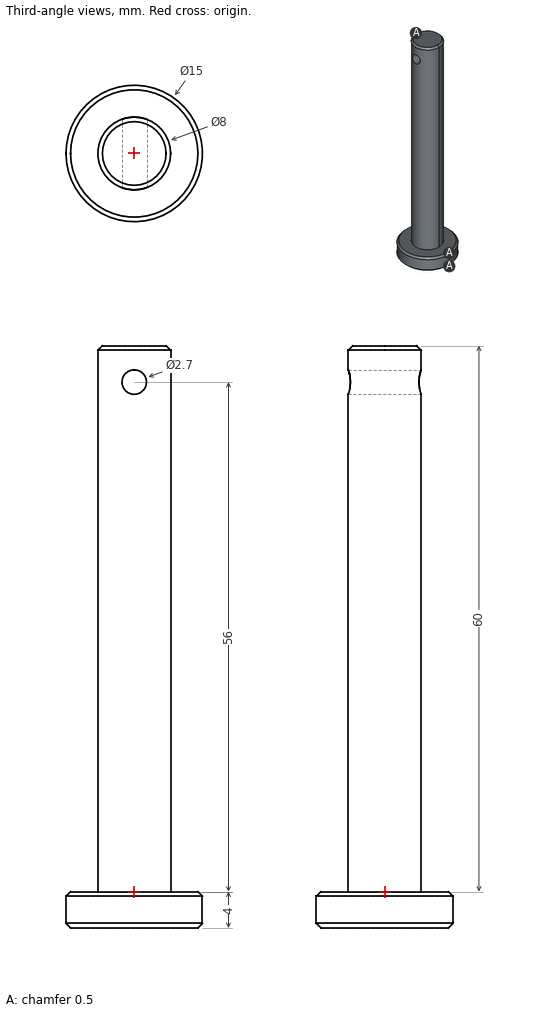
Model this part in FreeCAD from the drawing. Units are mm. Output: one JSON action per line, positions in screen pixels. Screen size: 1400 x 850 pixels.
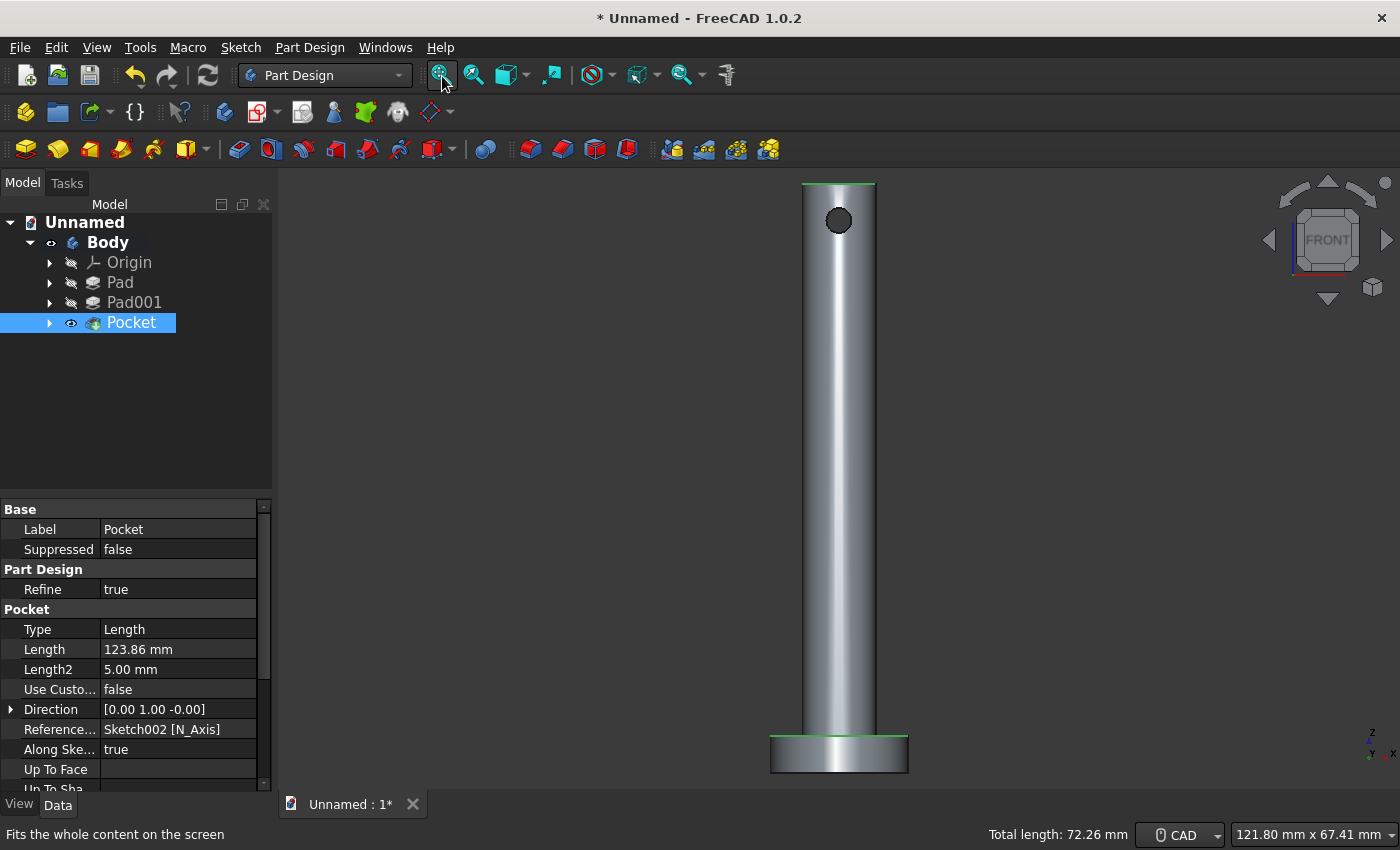
{"action": "key", "text": "3"}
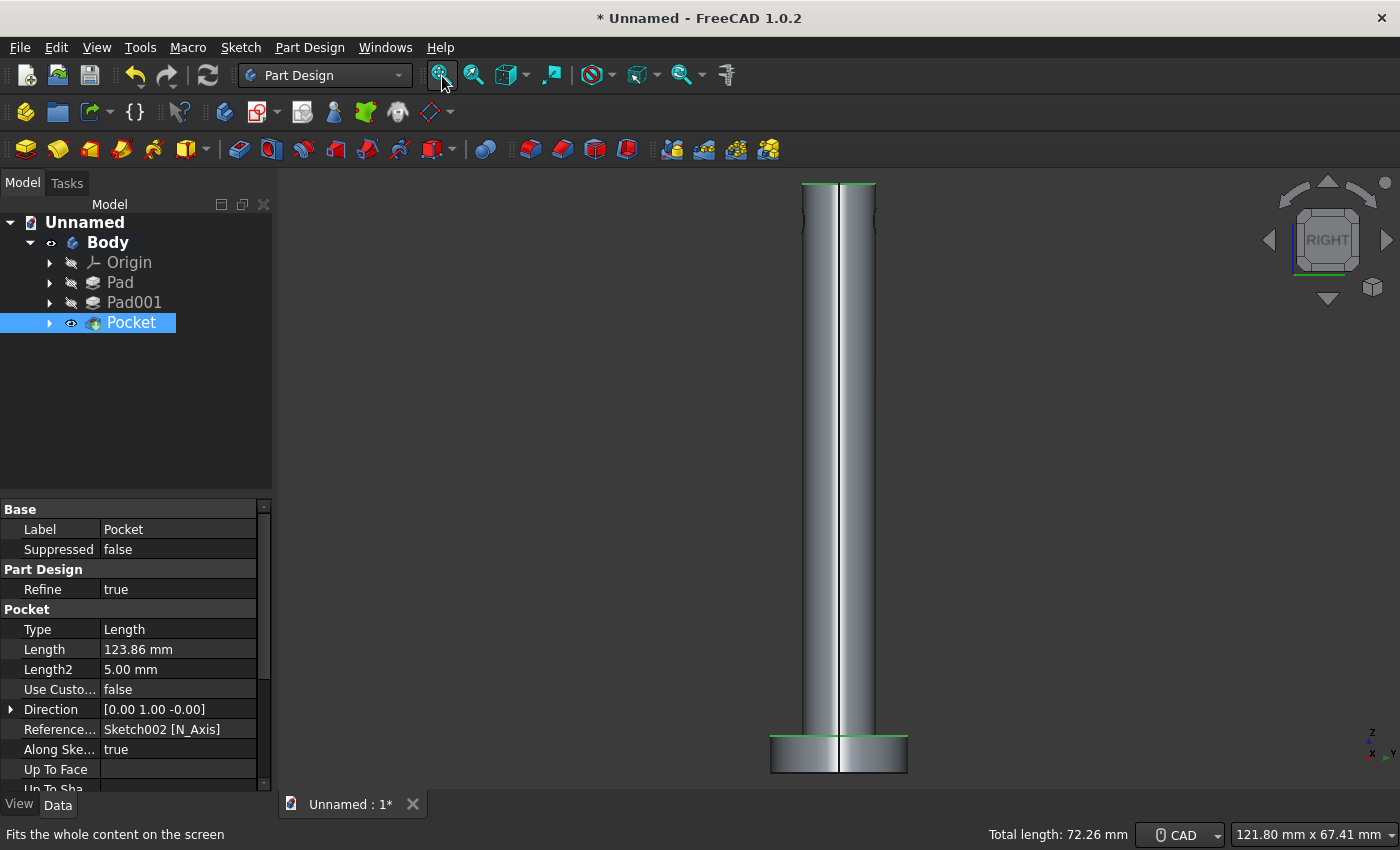
{"action": "key", "text": "5"}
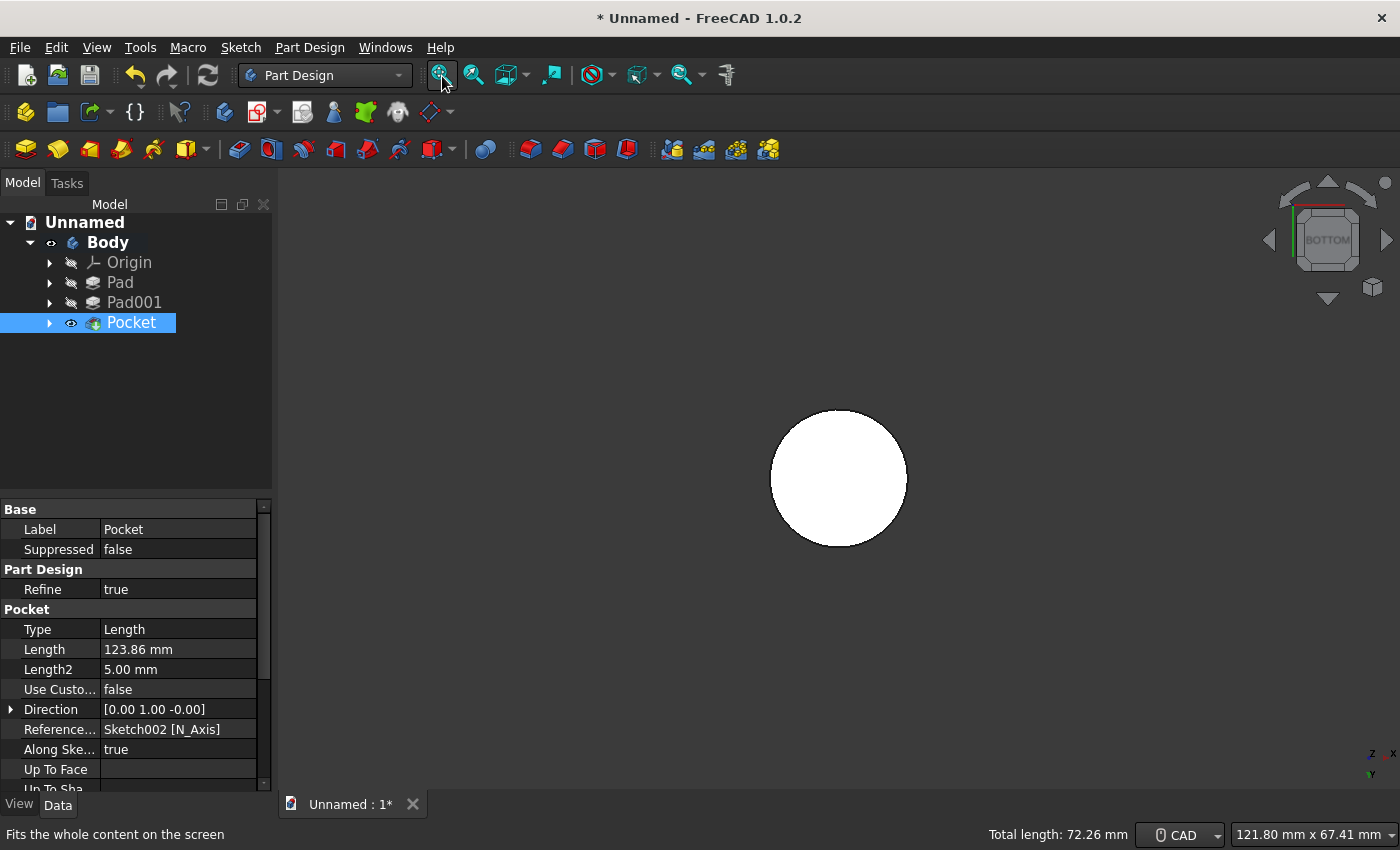
{"action": "left_click", "coordinate": [442, 76]}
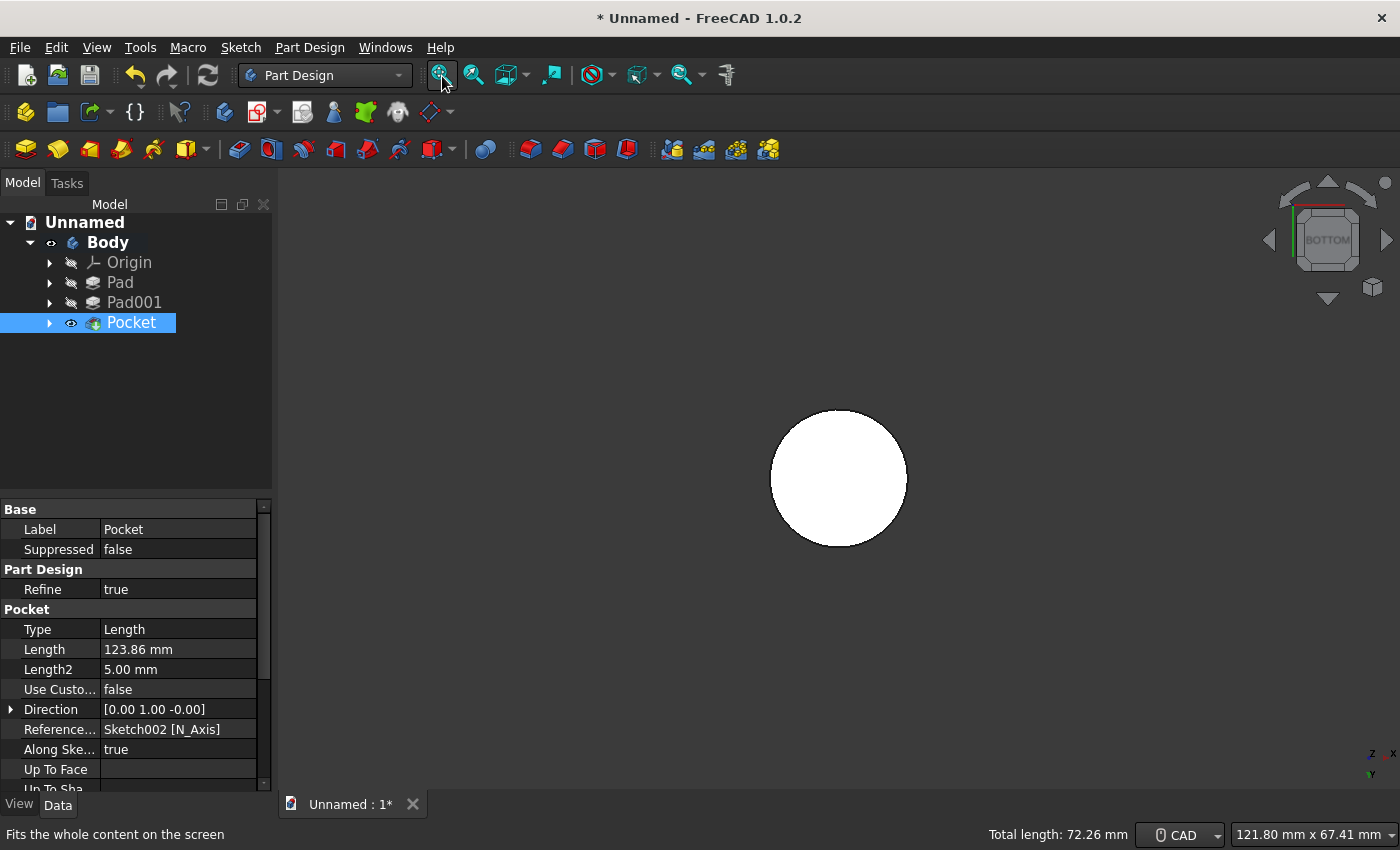
{"action": "left_click", "coordinate": [770, 477], "text": "ctrl"}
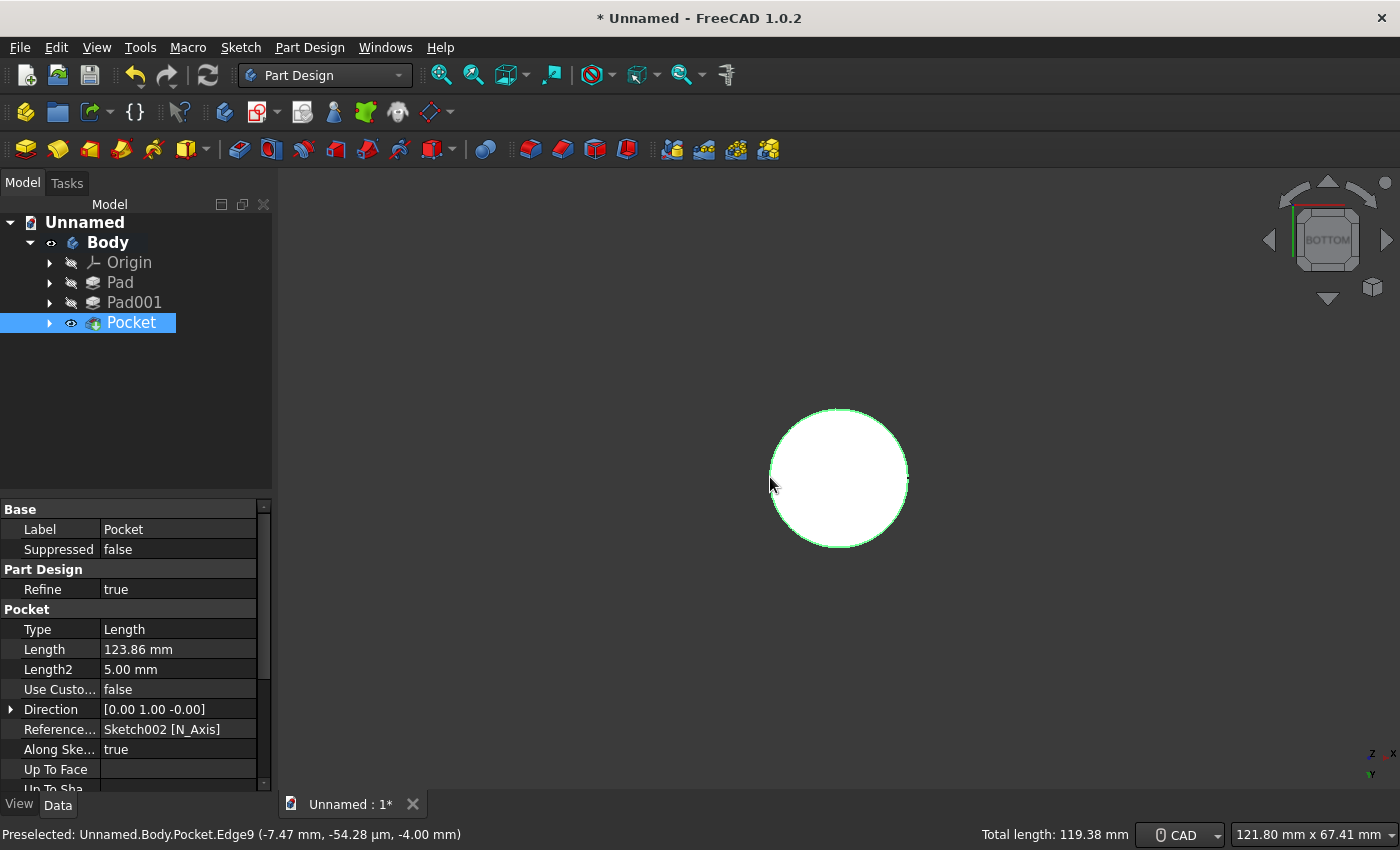
{"action": "left_click", "coordinate": [564, 150]}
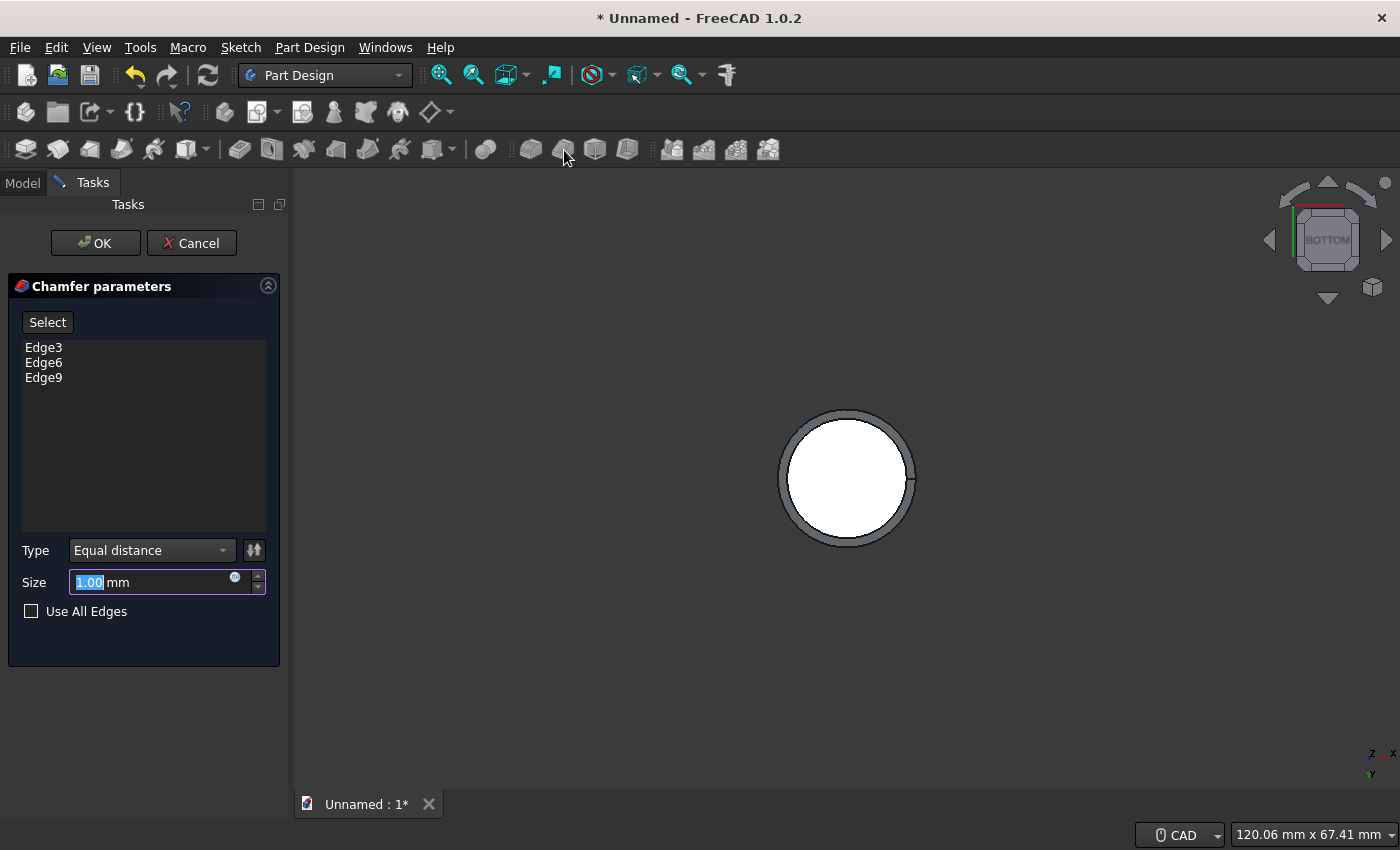
{"action": "type", "text": "0.5"}
{"action": "key", "text": "Tab"}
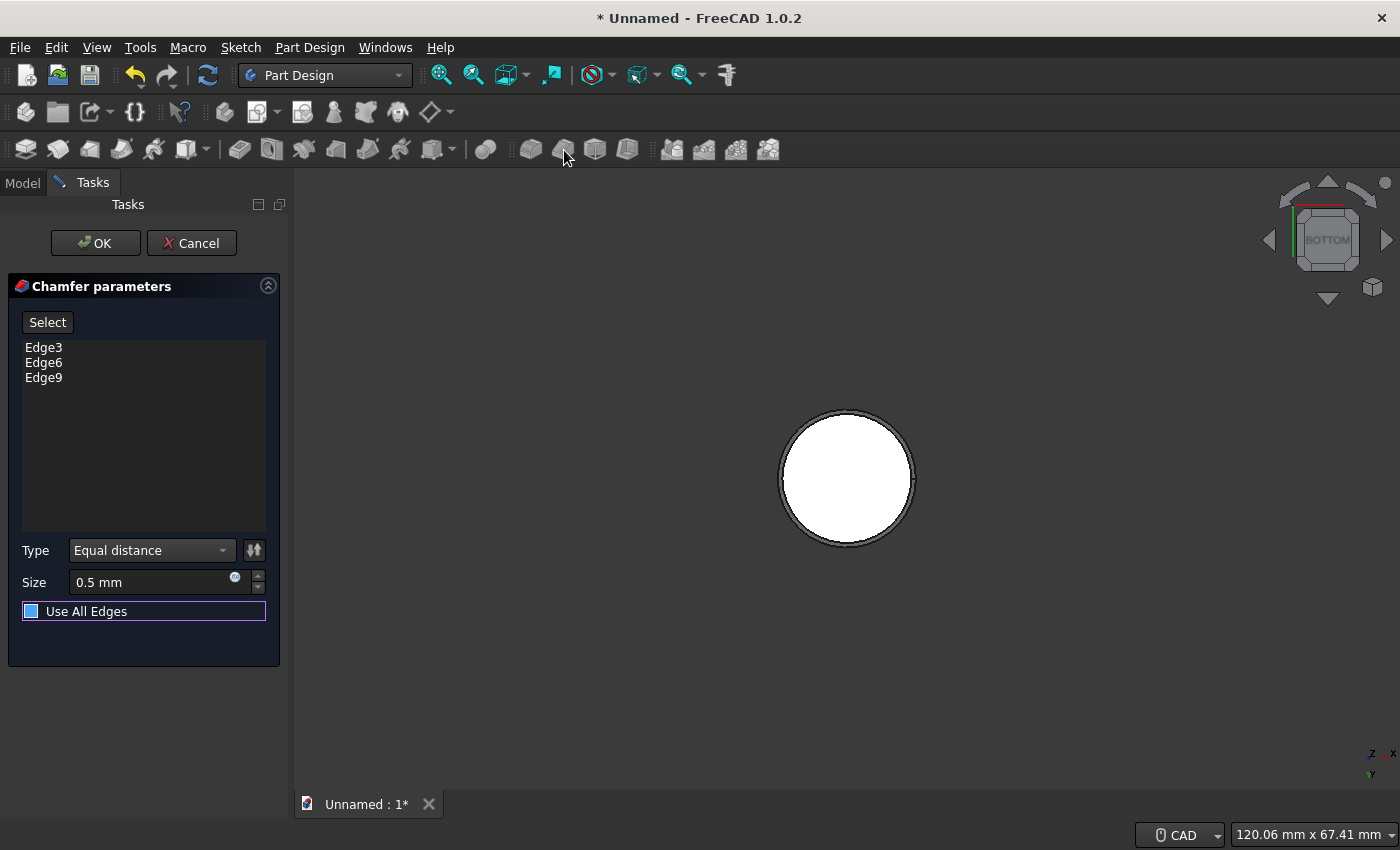
{"action": "left_click", "coordinate": [96, 243]}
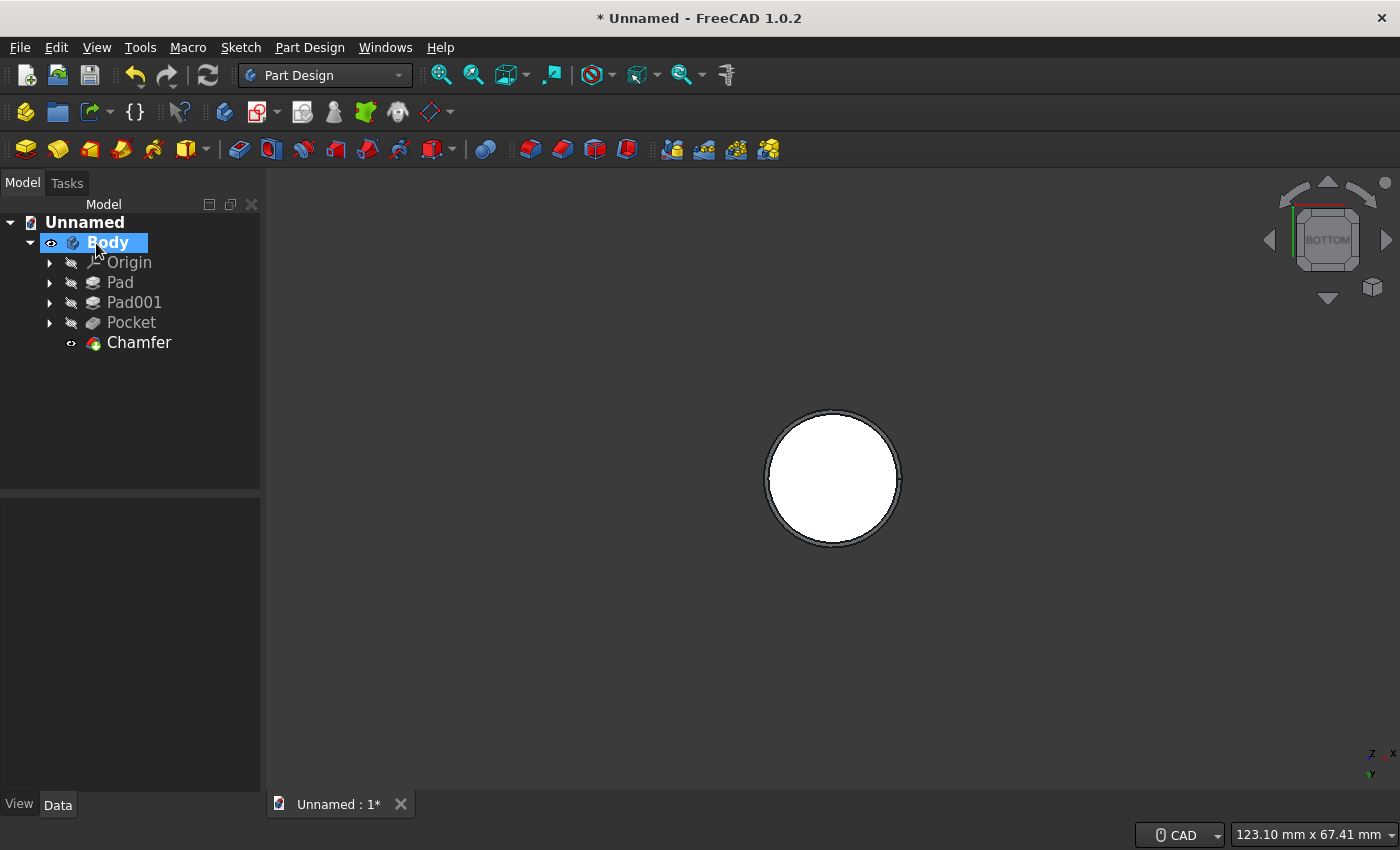
{"action": "key", "text": "0"}